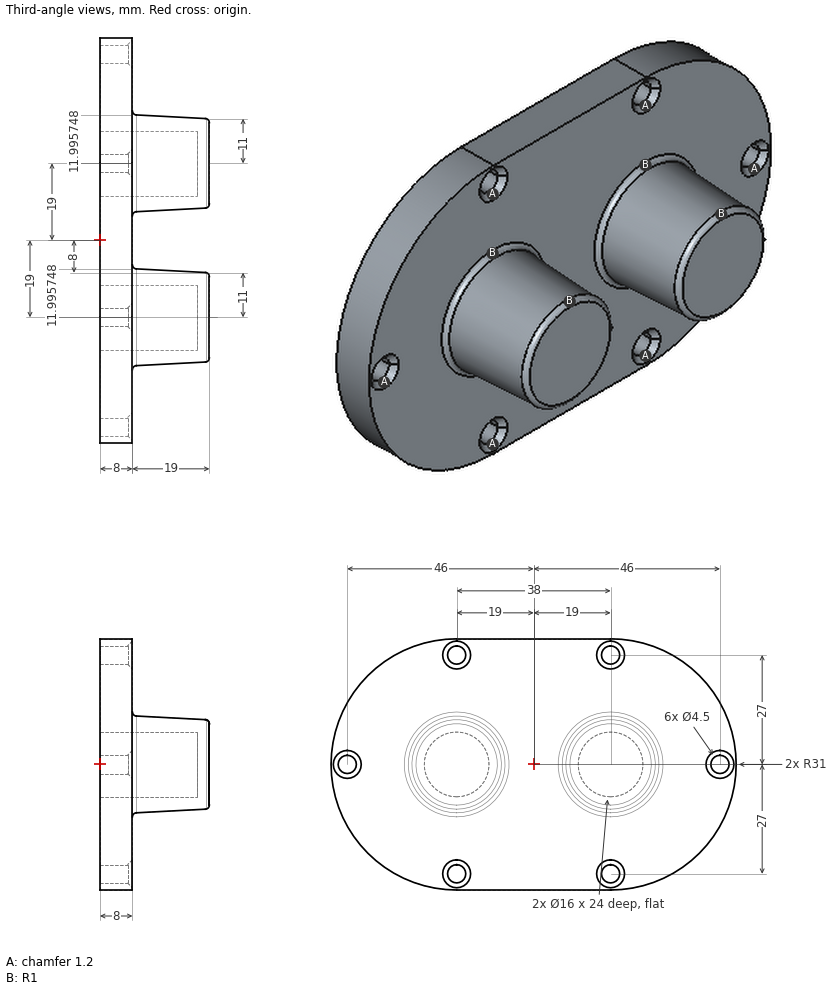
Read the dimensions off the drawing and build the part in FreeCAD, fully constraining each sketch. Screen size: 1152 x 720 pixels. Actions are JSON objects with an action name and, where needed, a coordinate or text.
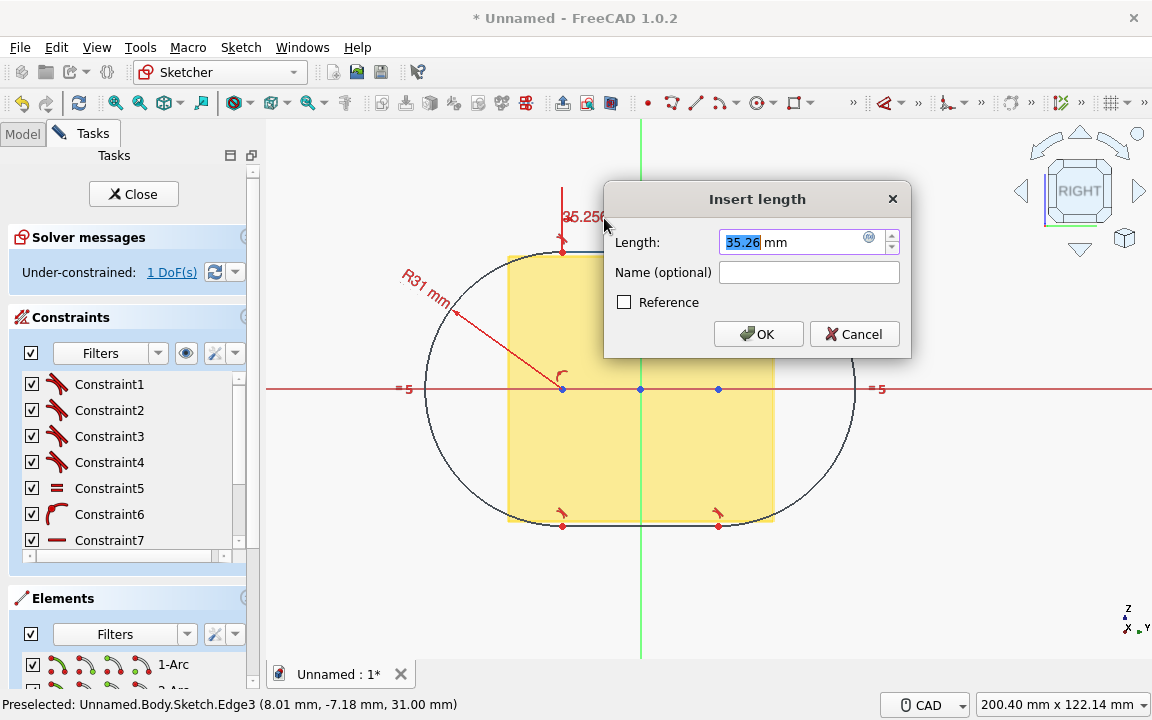
{"action": "type", "text": "38"}
{"action": "key", "text": "Return"}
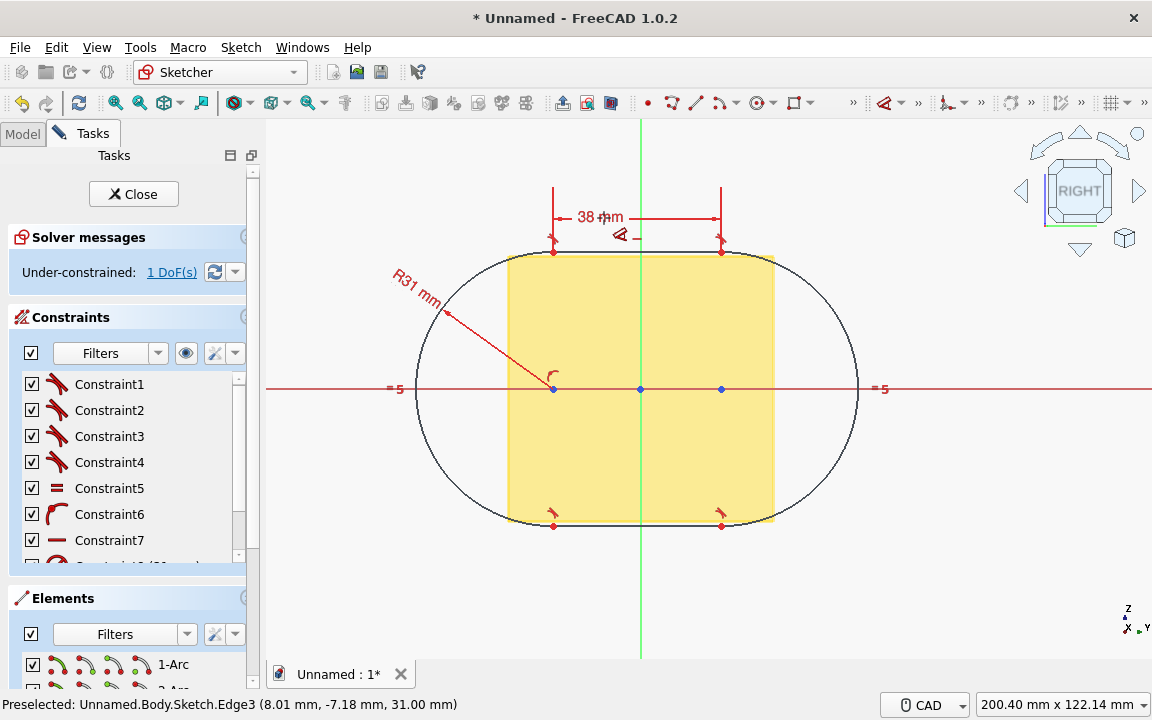
{"action": "left_click", "coordinate": [553, 252]}
{"action": "left_click", "coordinate": [597, 423]}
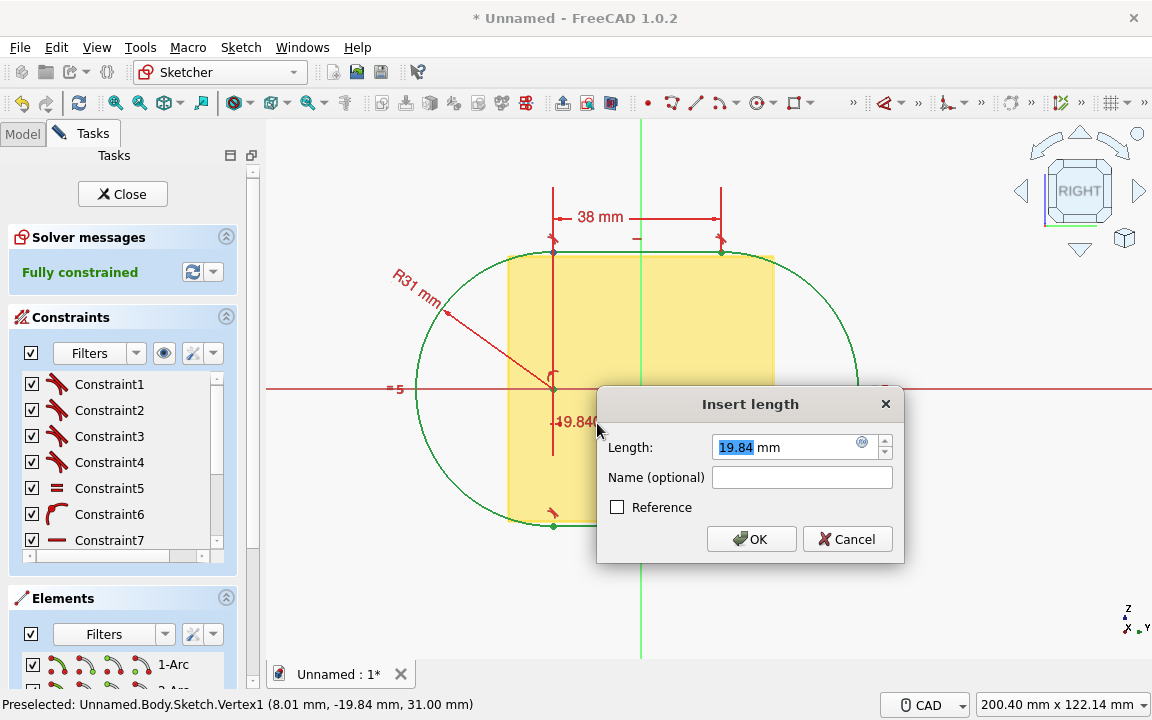
{"action": "type", "text": "19"}
{"action": "key", "text": "Return"}
{"action": "key", "text": "Escape"}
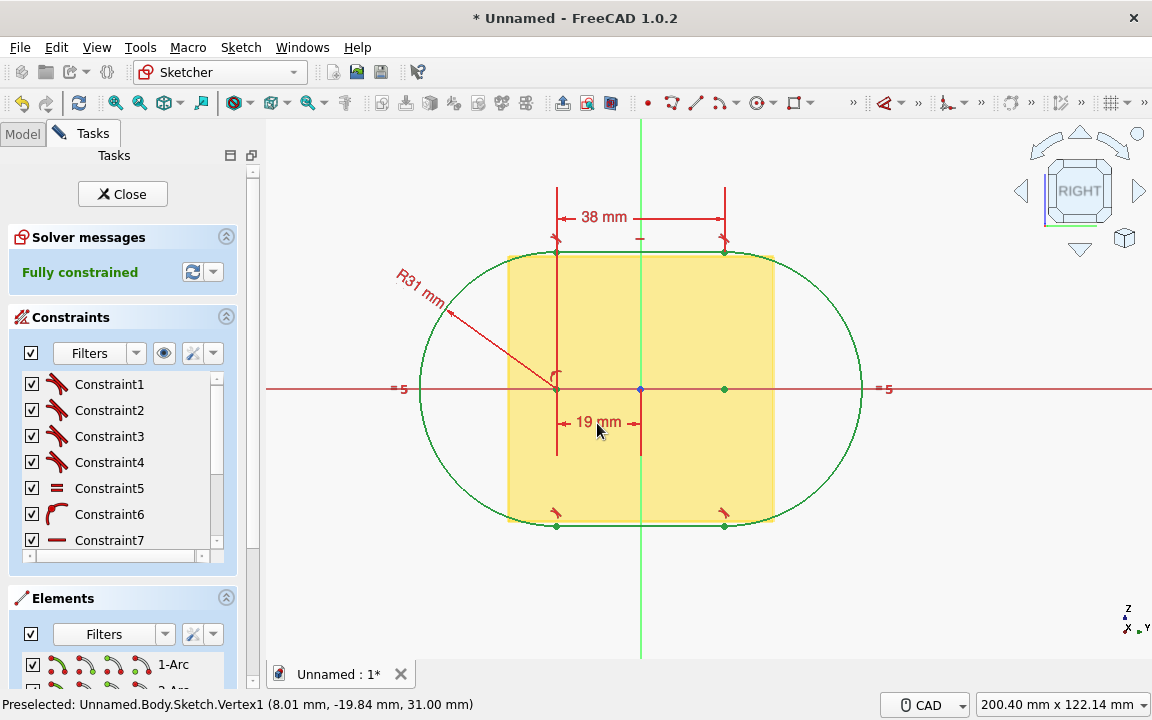
{"action": "left_click", "coordinate": [123, 194]}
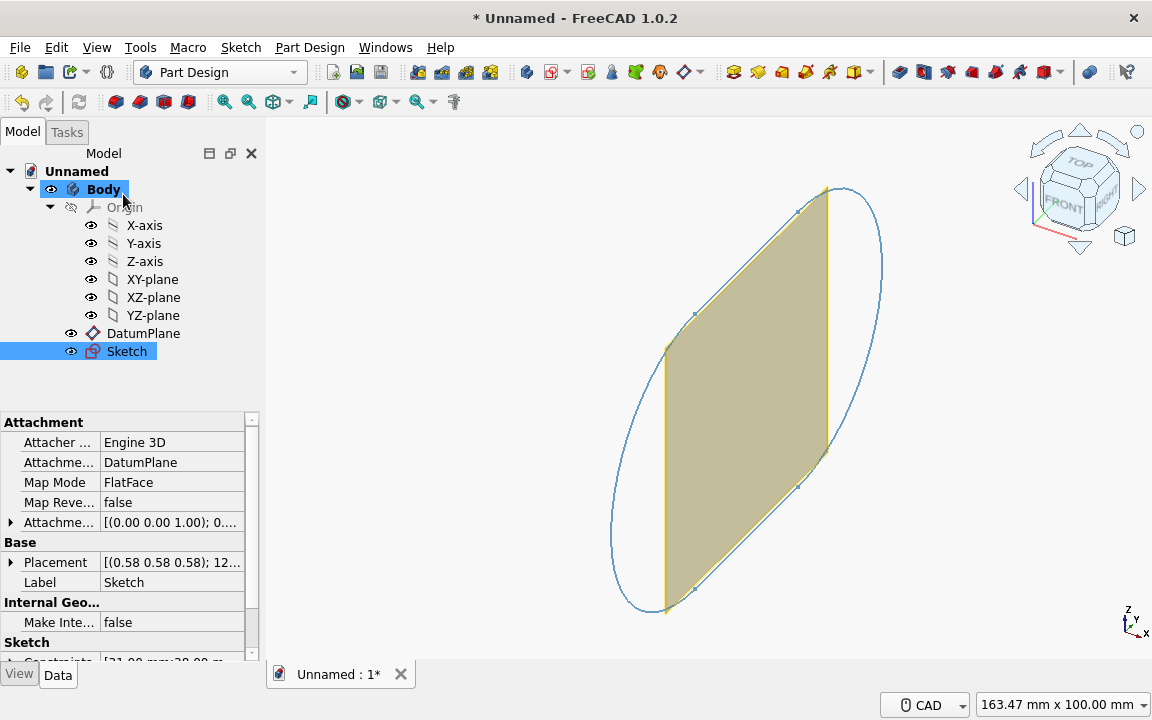
{"action": "left_click", "coordinate": [734, 72]}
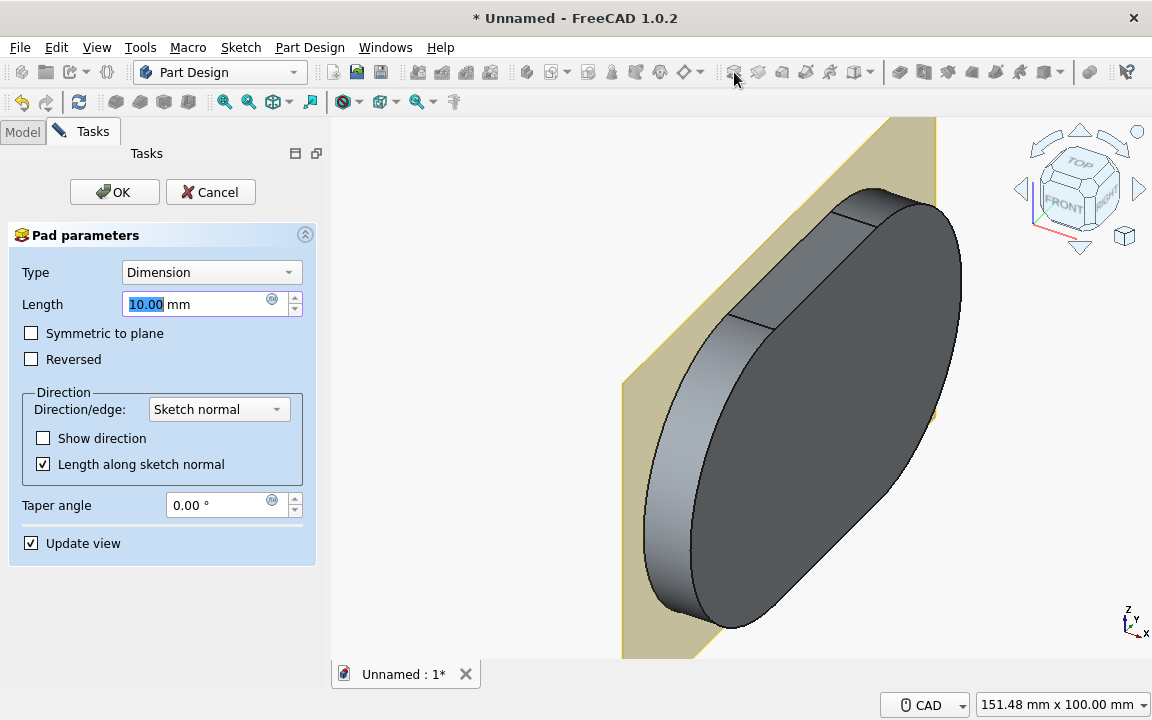
{"action": "type", "text": "8"}
{"action": "key", "text": "Tab"}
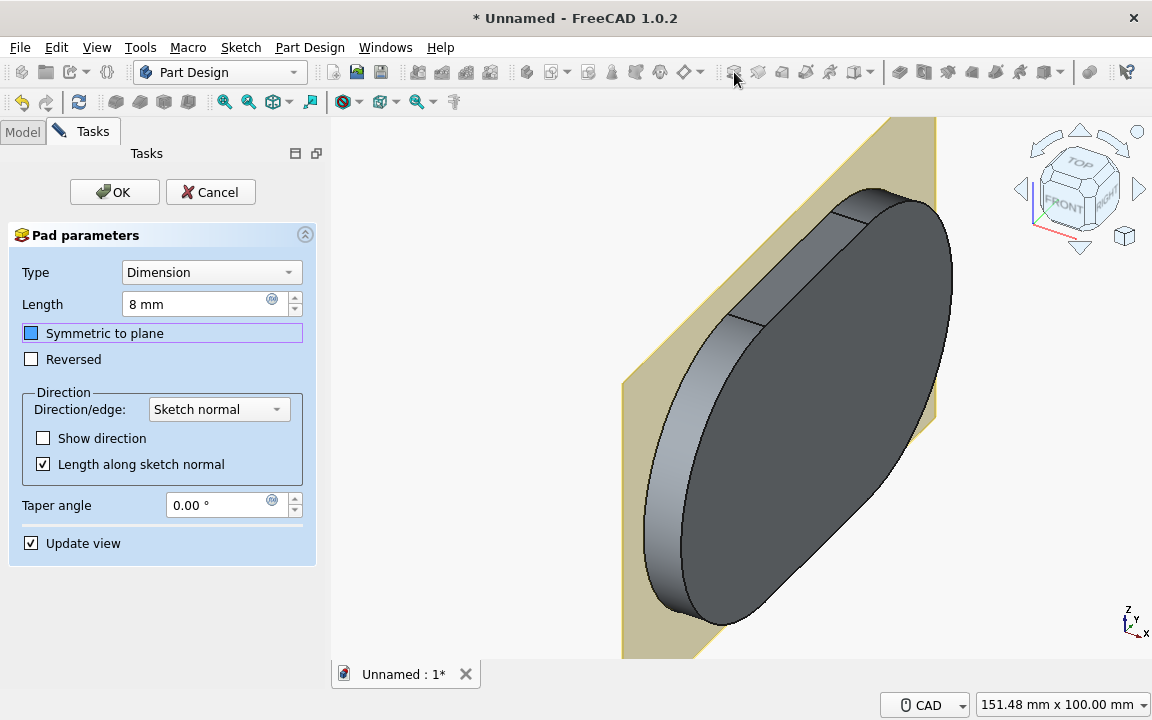
{"action": "left_click", "coordinate": [30, 359]}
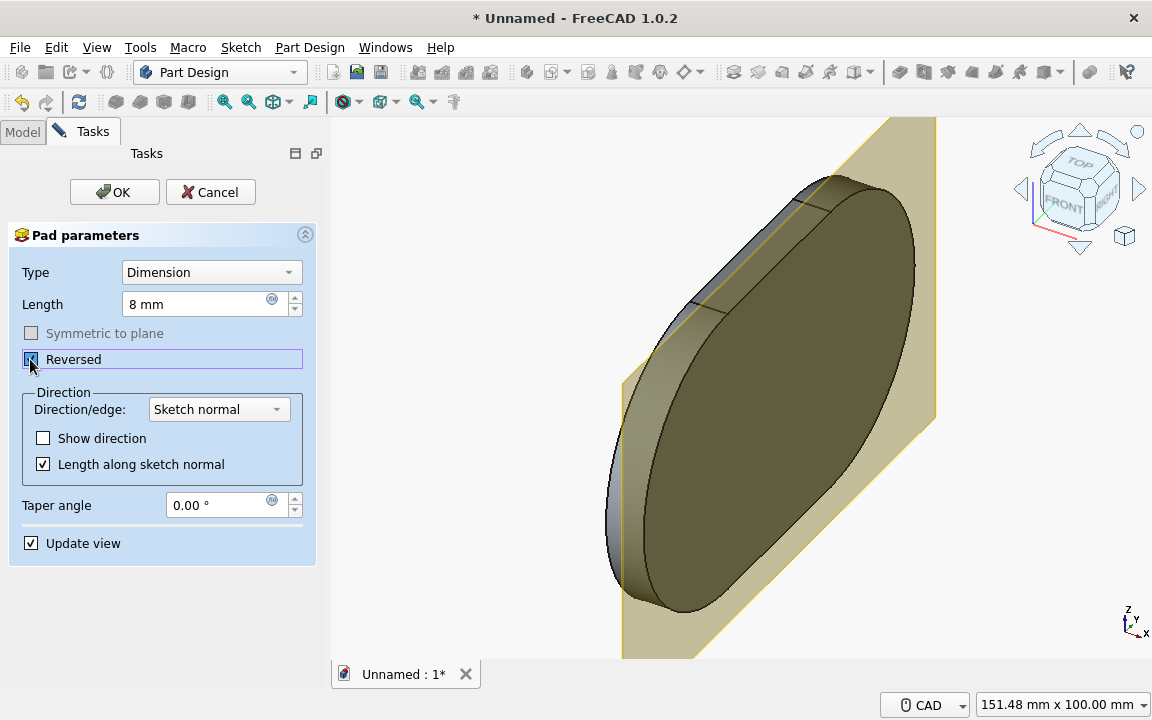
{"action": "left_click", "coordinate": [115, 192]}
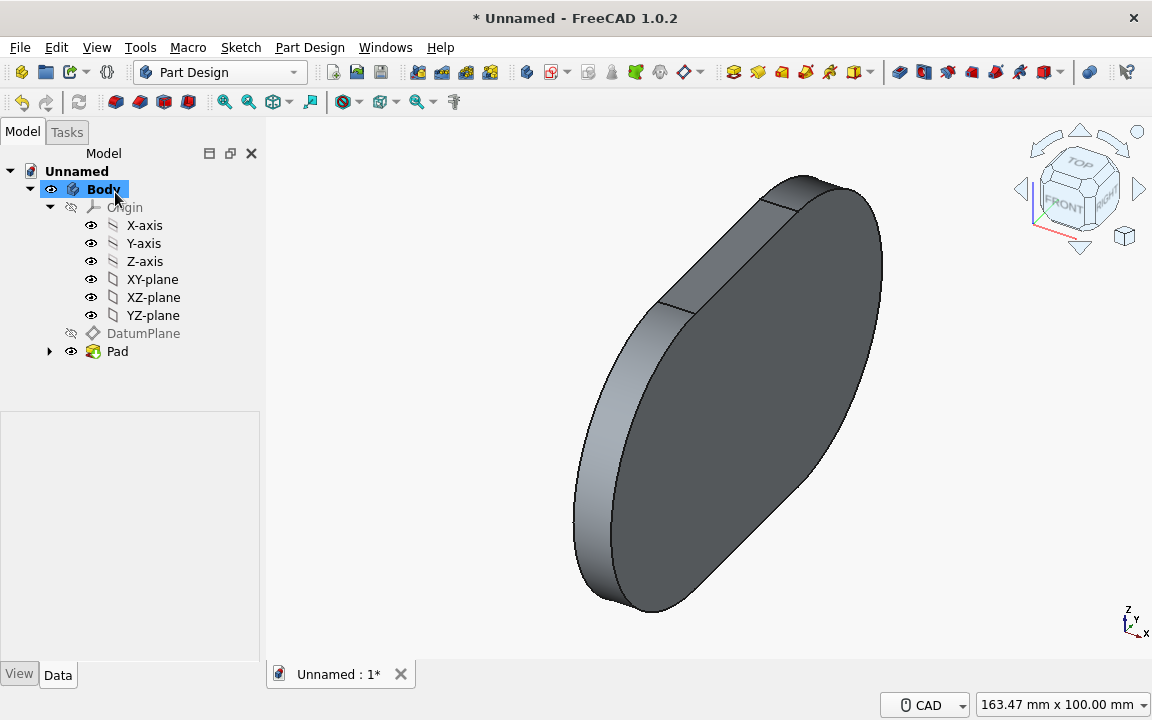
{"action": "left_click", "coordinate": [226, 102]}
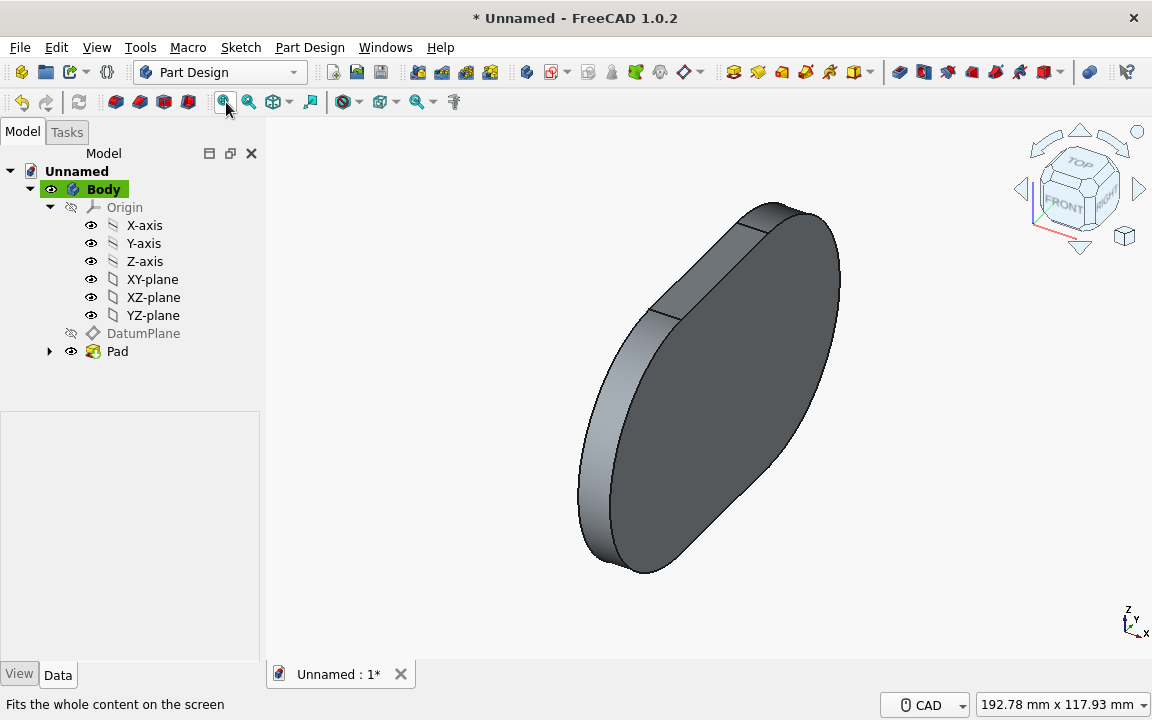
{"action": "left_click", "coordinate": [552, 72]}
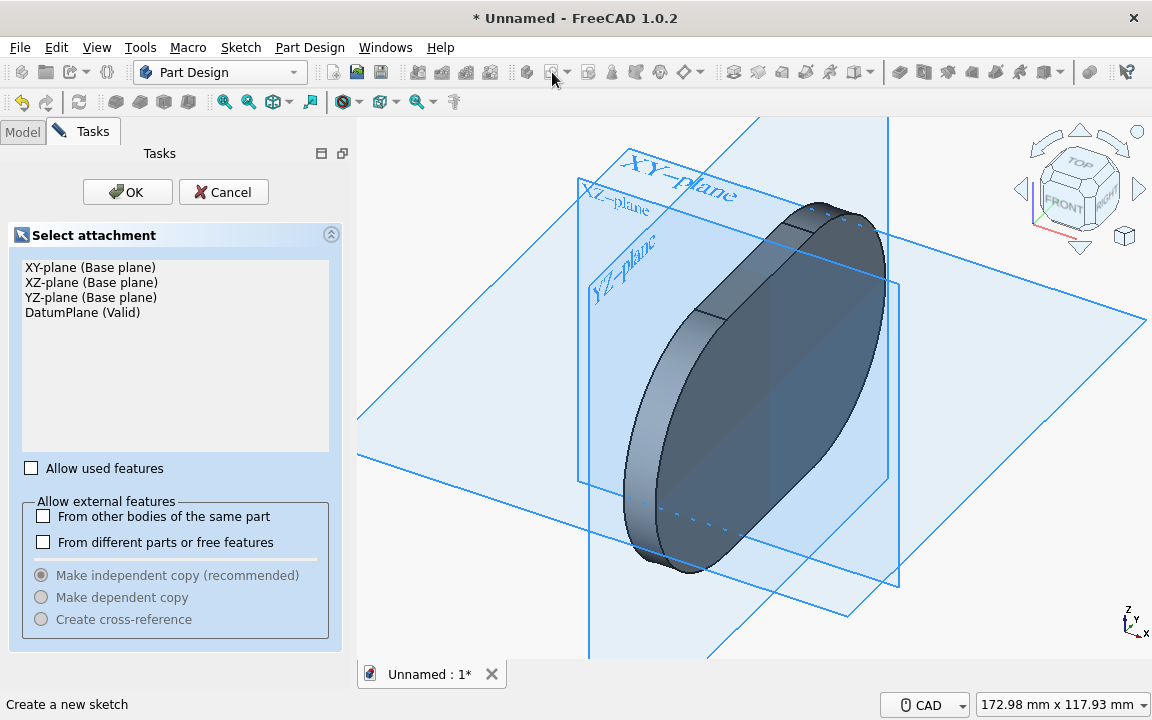
{"action": "left_click", "coordinate": [82, 268]}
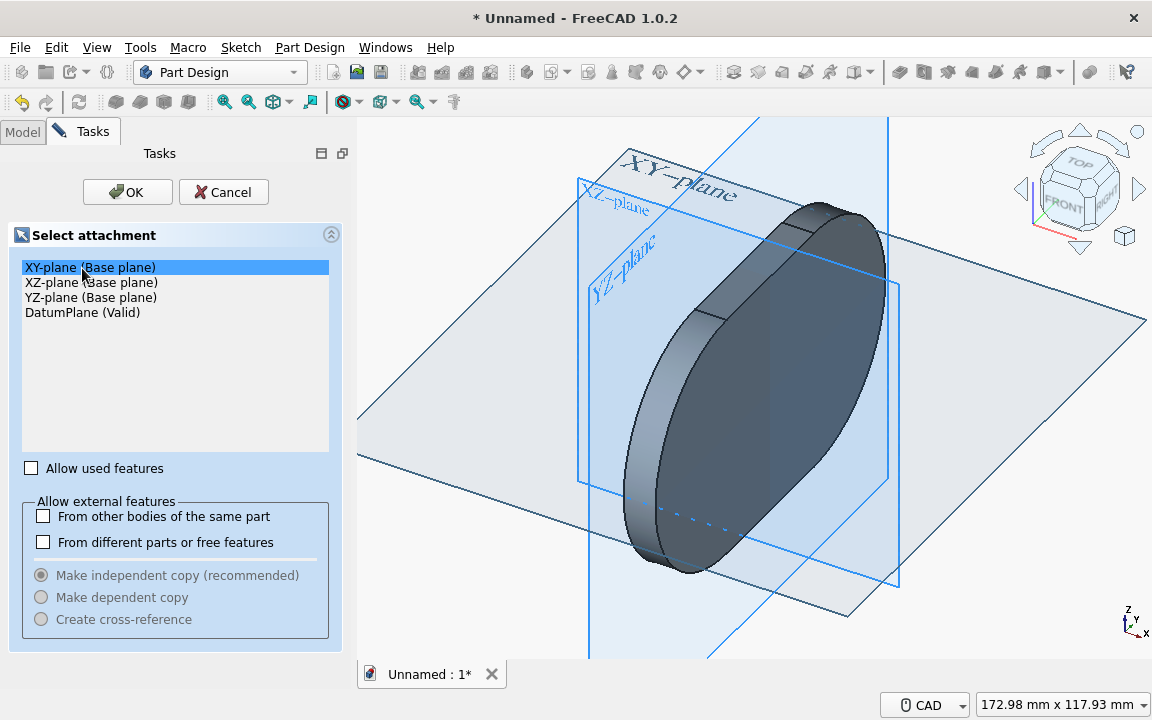
{"action": "left_click", "coordinate": [128, 192]}